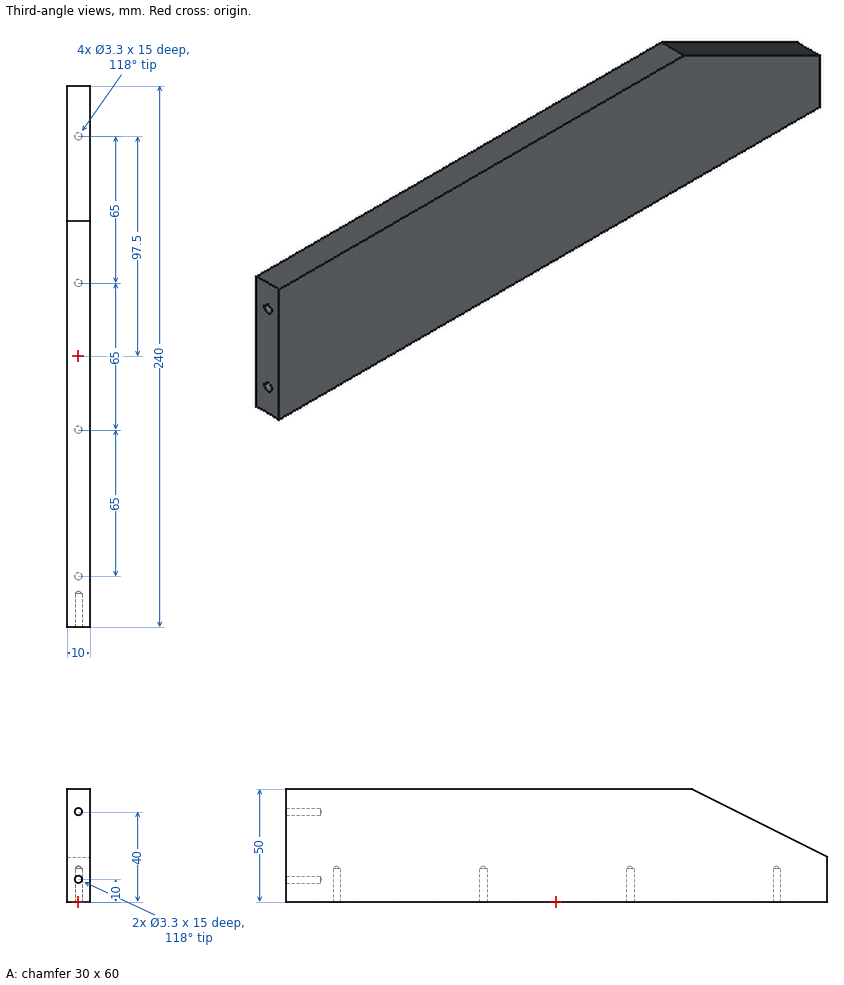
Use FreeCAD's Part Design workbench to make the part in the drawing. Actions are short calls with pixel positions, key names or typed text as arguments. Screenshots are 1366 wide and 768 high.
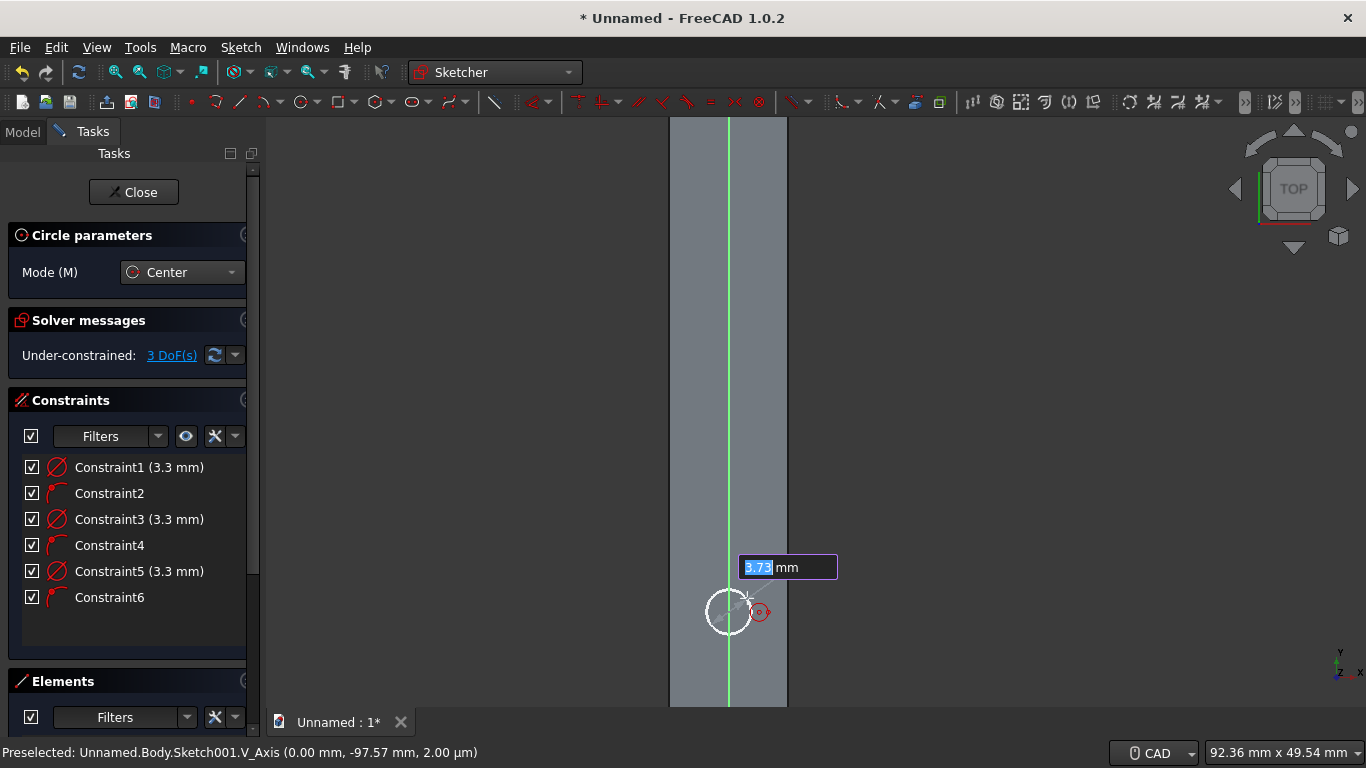
text(3.3)
key(Return)
key(Escape)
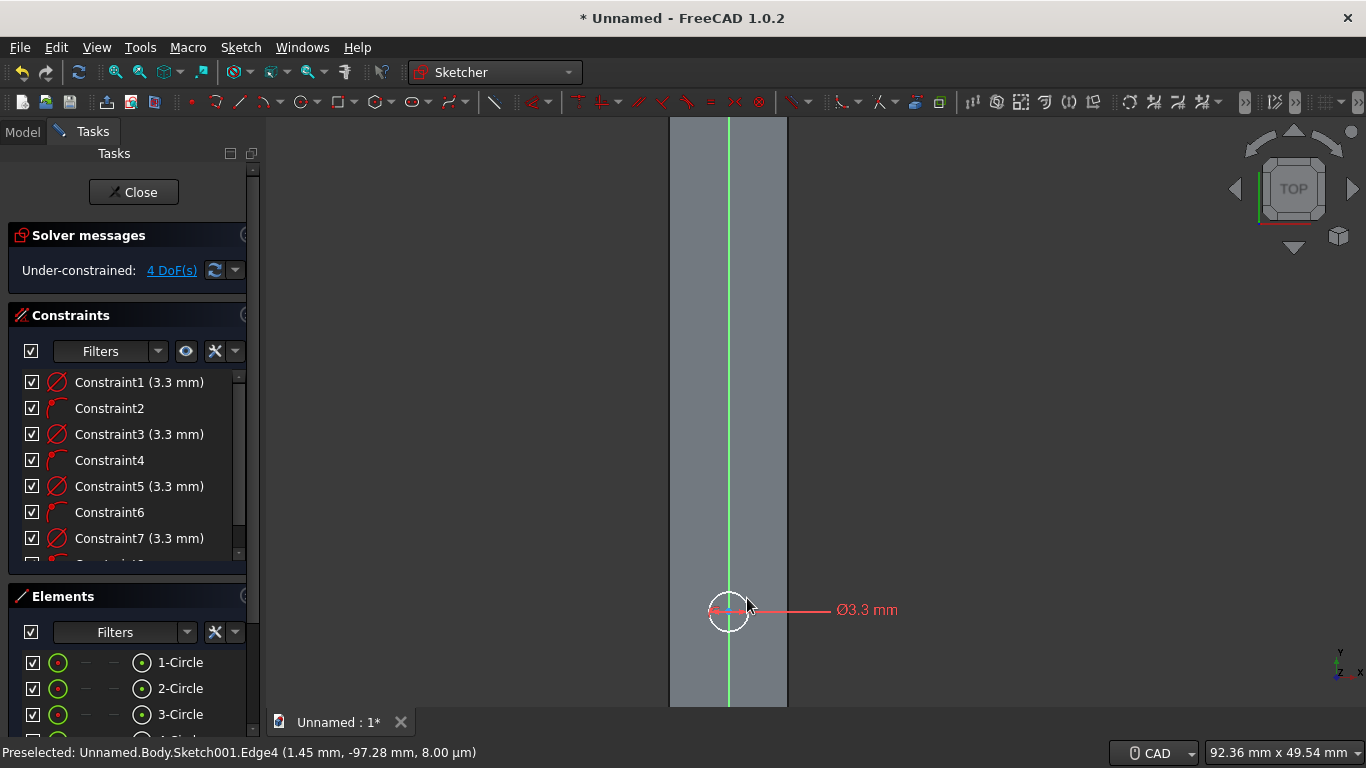
click(532, 102)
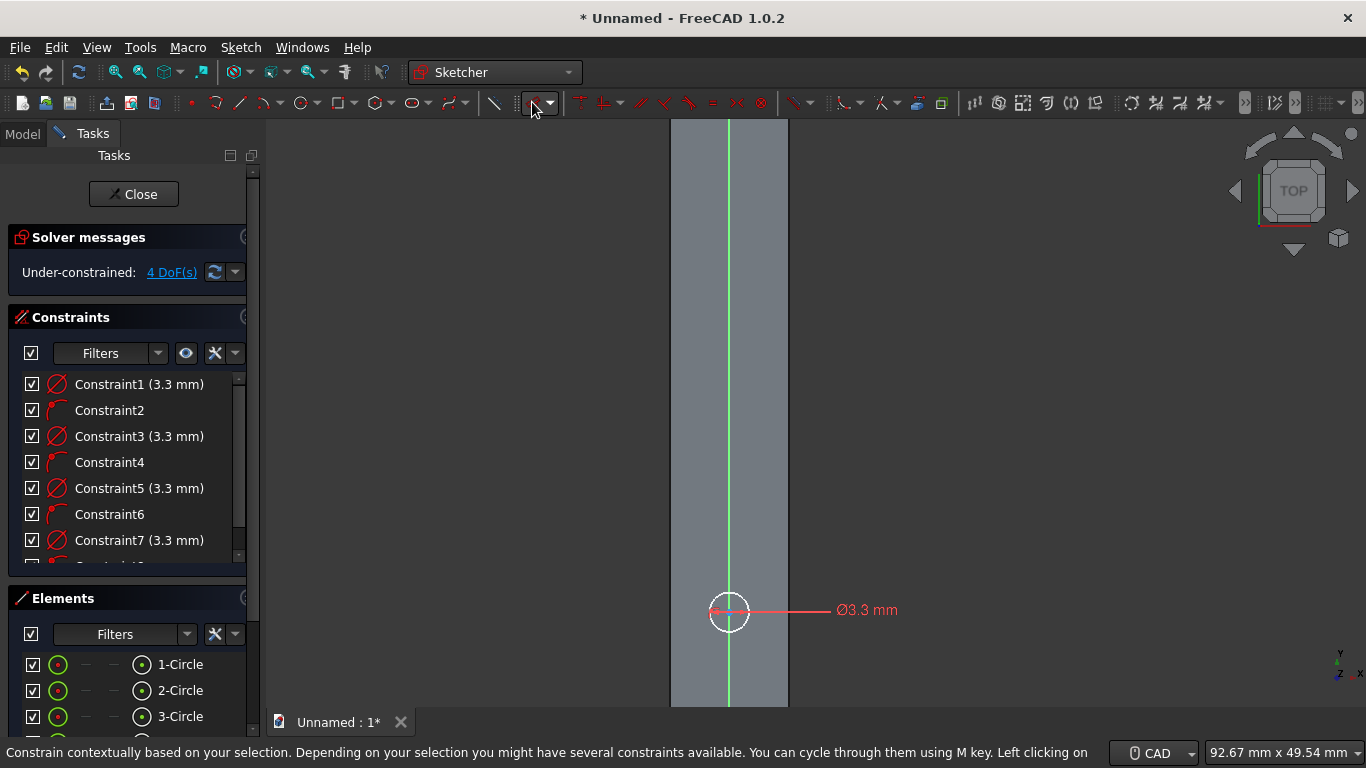
scroll(751, 604, down, 9)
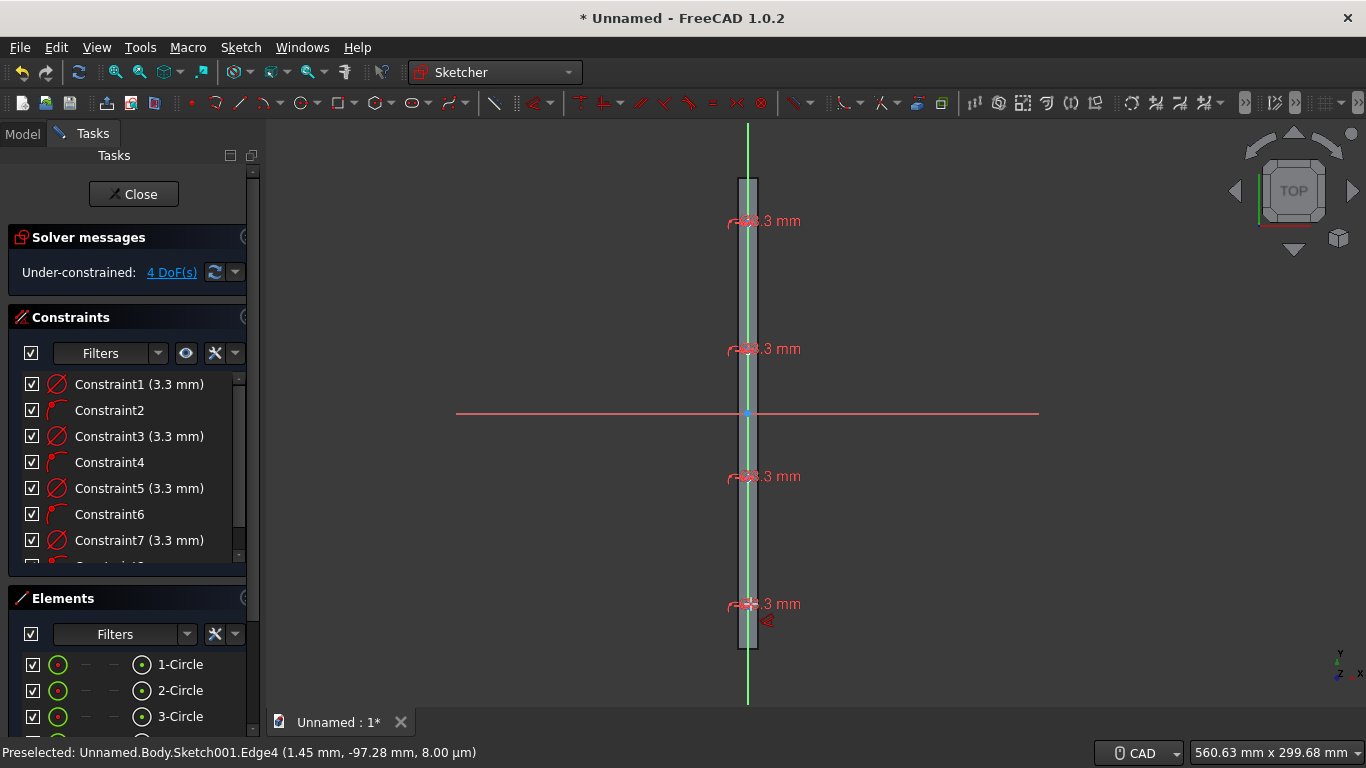
click(748, 223)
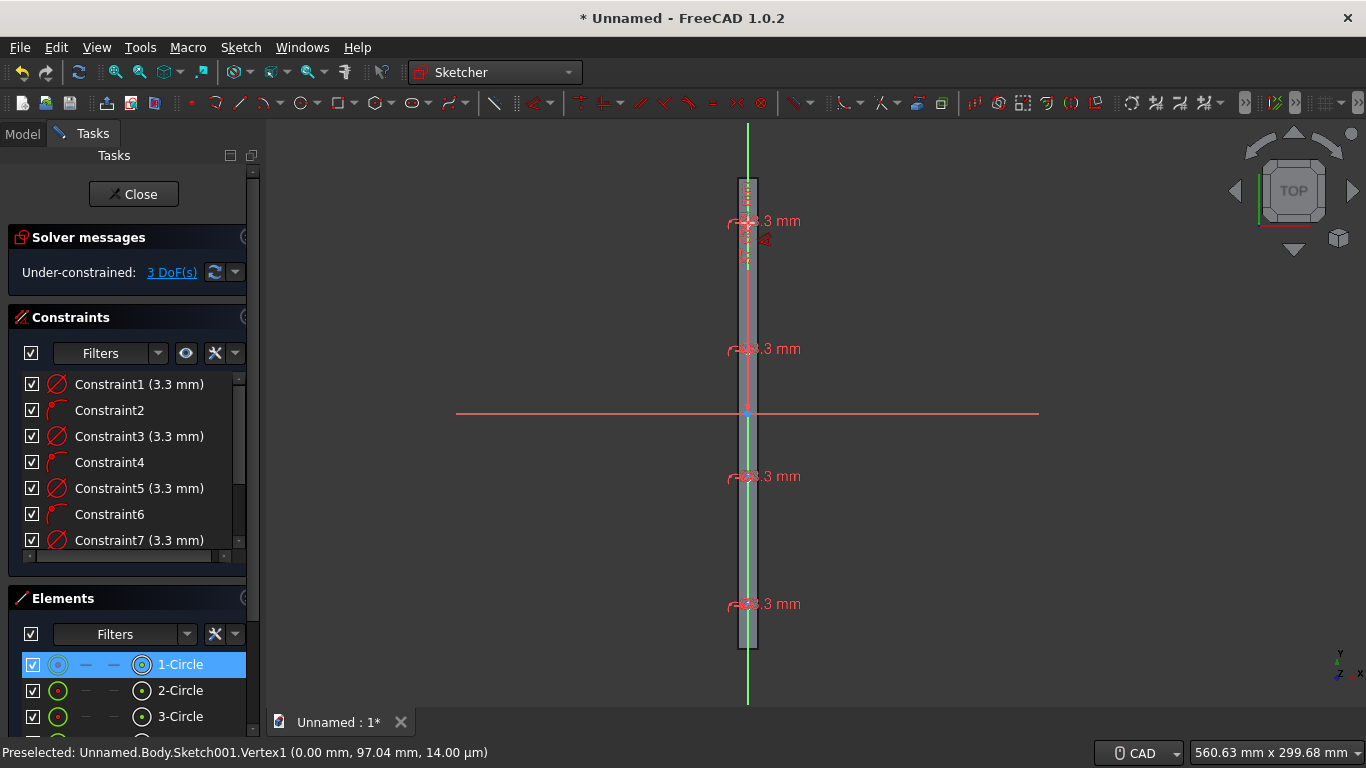
click(748, 351)
click(782, 287)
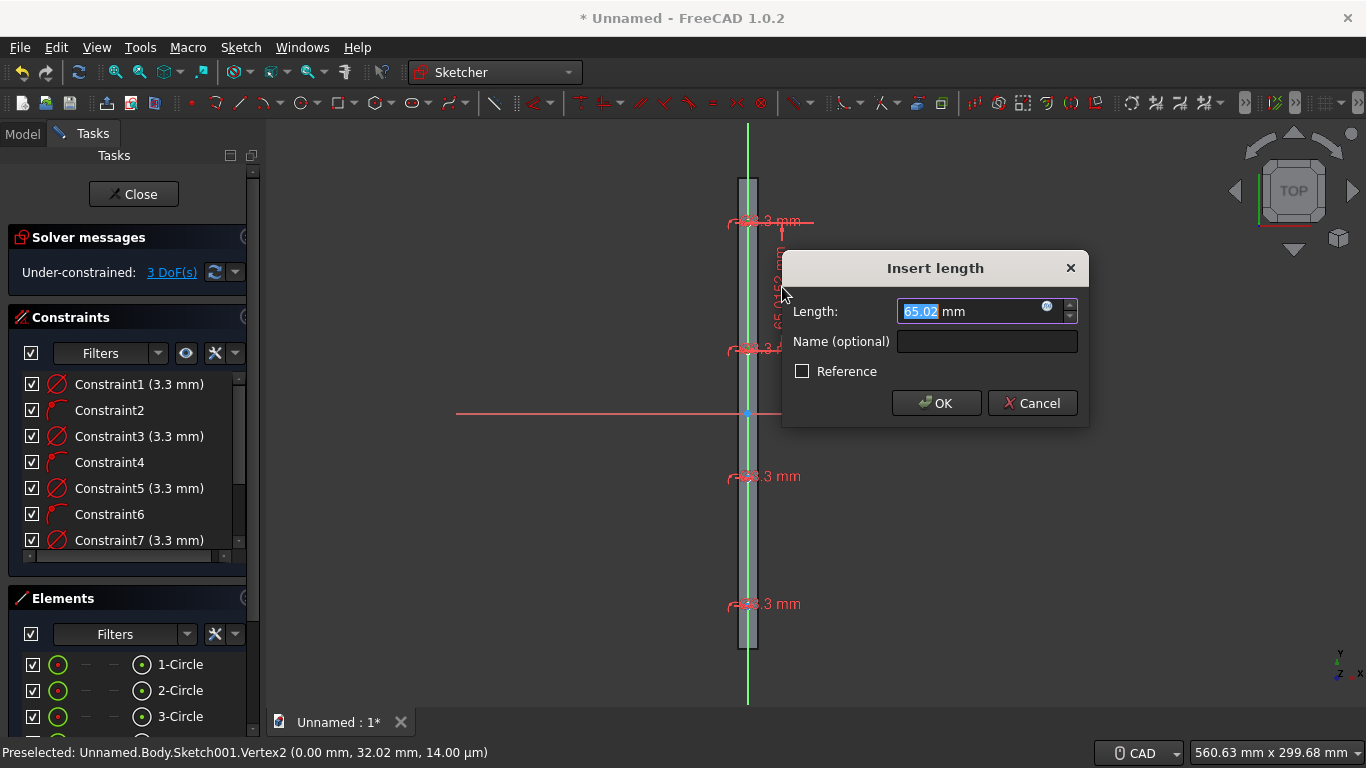
text(65)
key(Return)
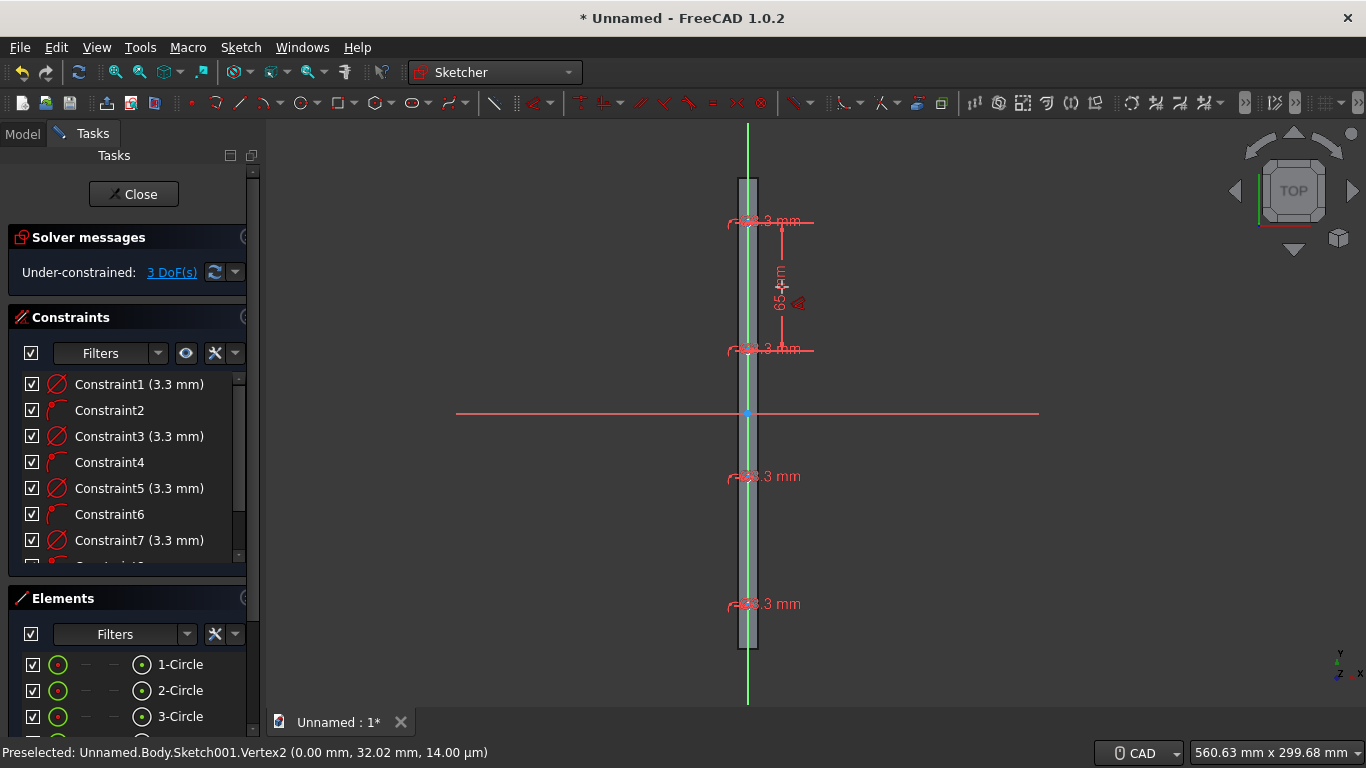
click(748, 351)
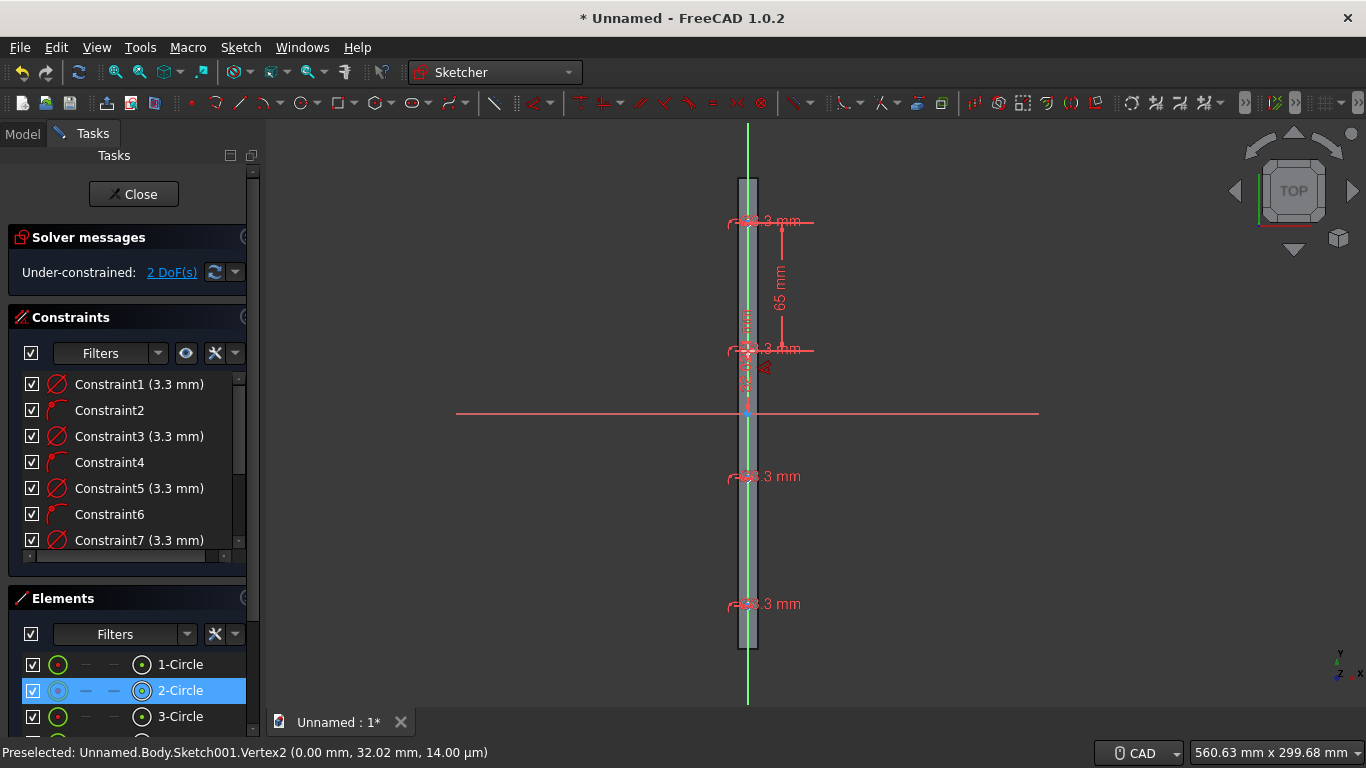
click(748, 478)
click(782, 385)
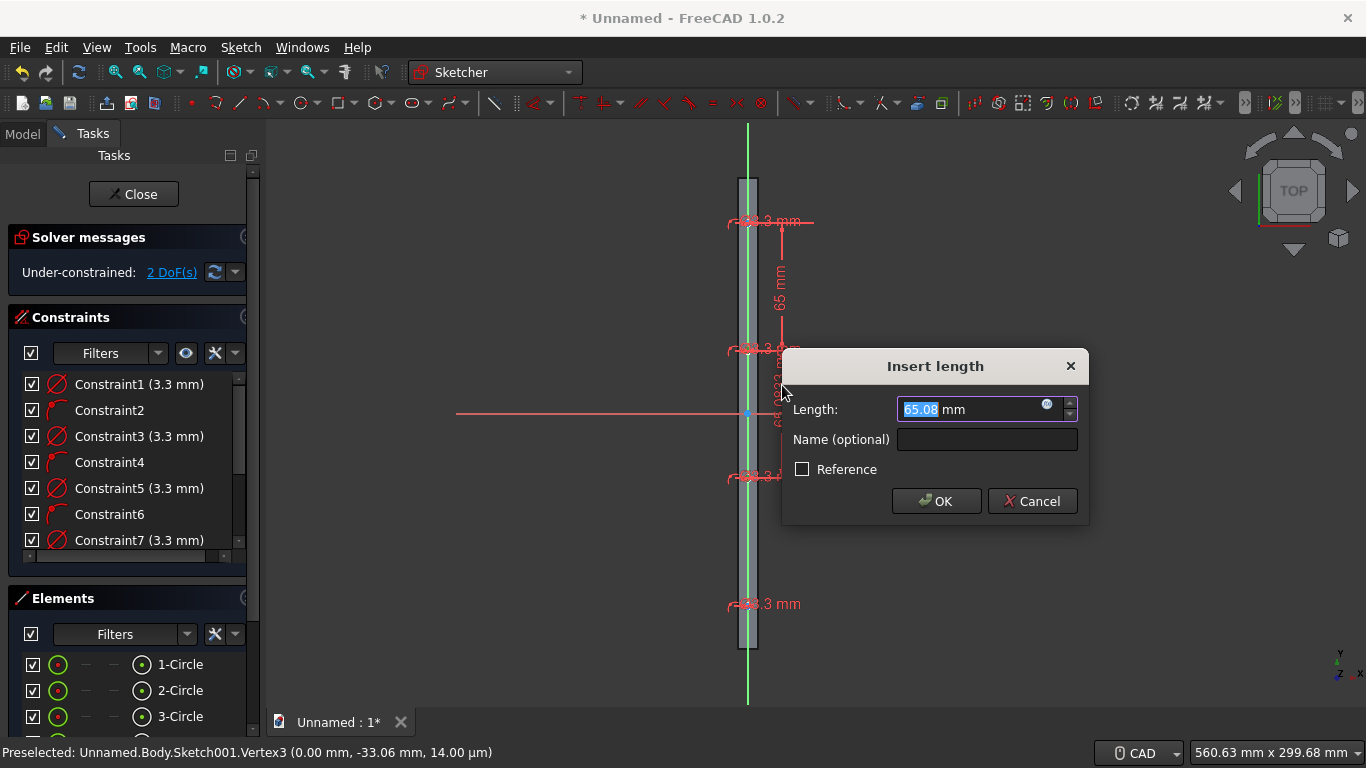
text(65)
key(Return)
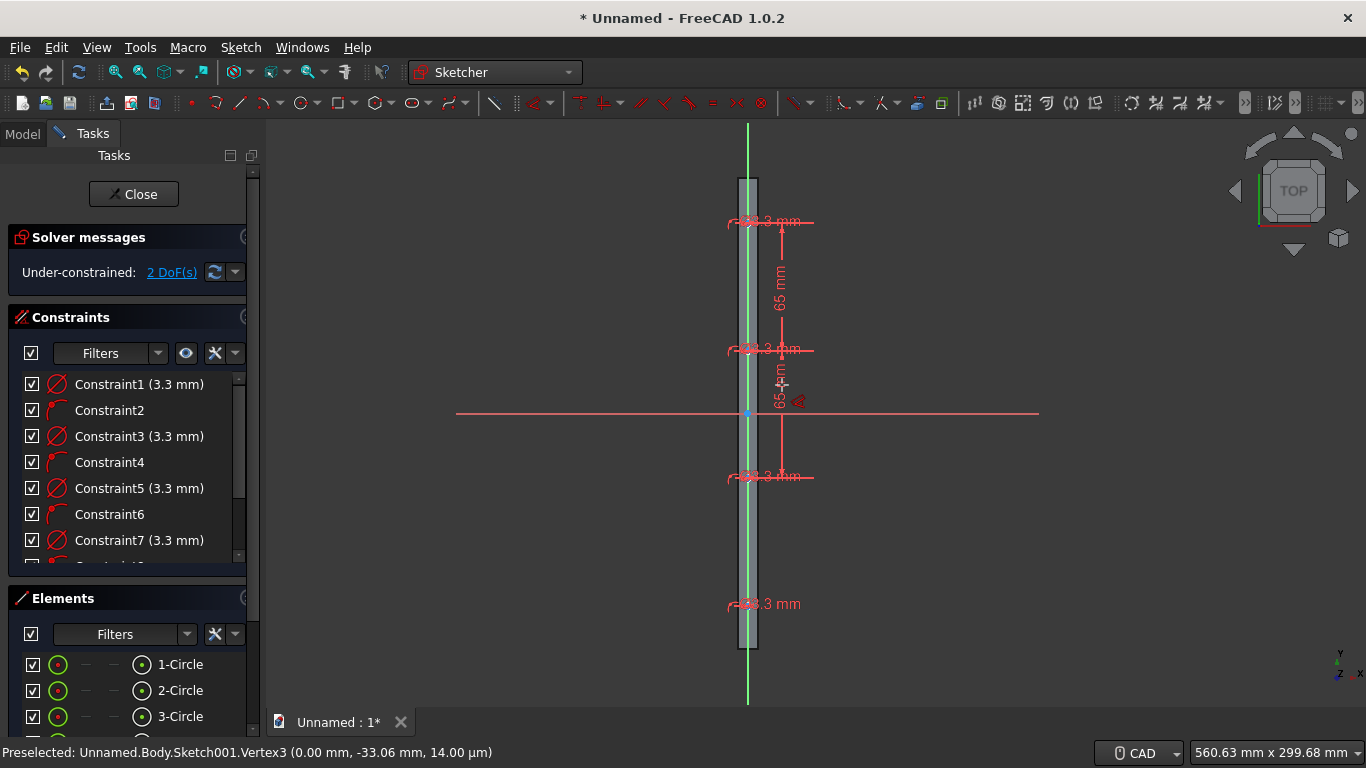
click(748, 478)